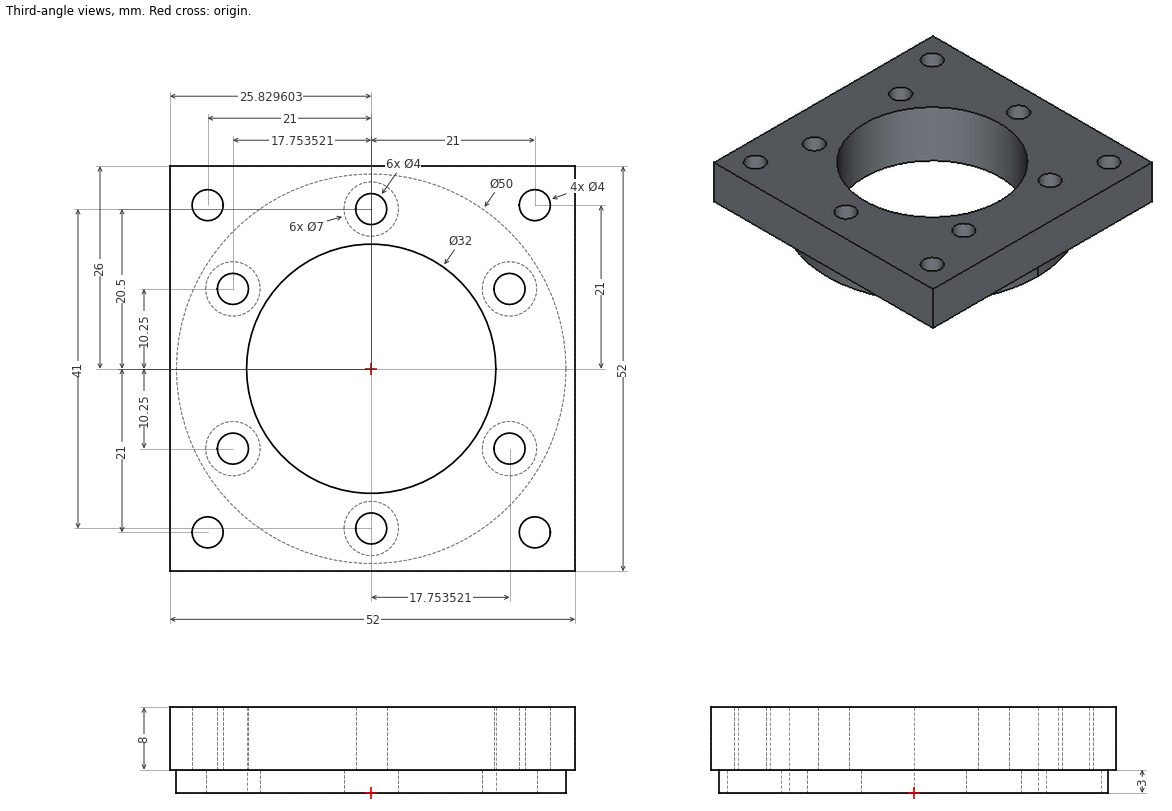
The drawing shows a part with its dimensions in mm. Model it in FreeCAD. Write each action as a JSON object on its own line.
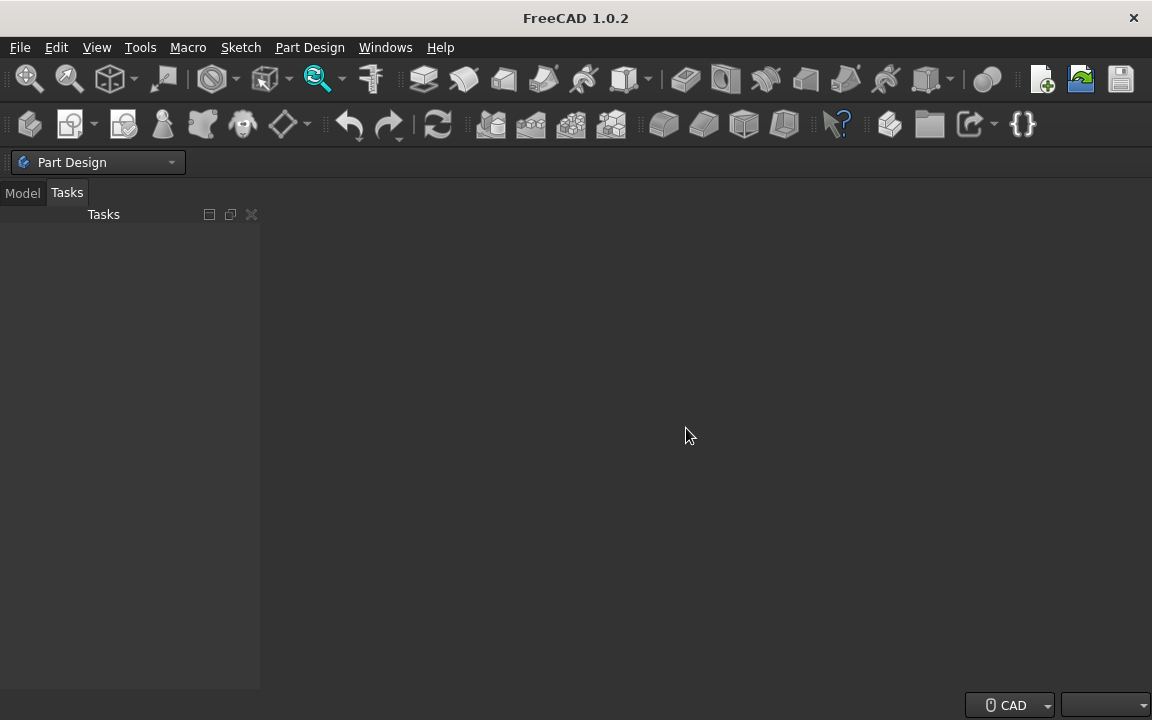
{"action": "key", "text": "ctrl+n"}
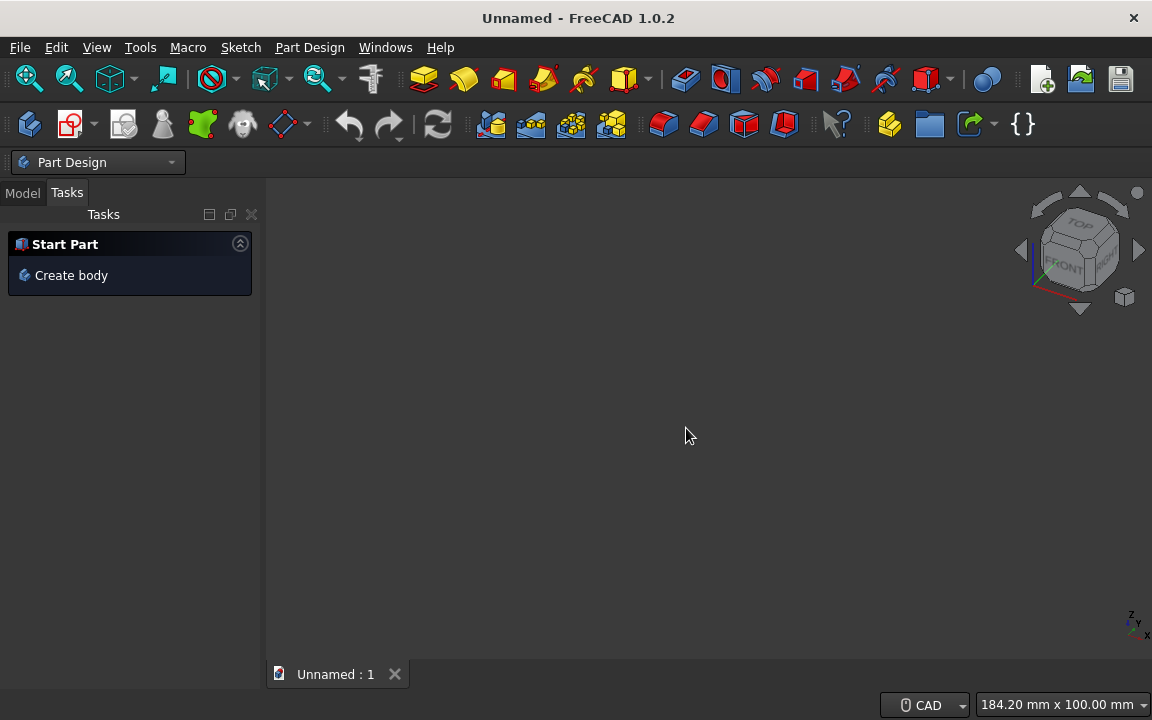
{"action": "left_click", "coordinate": [70, 124]}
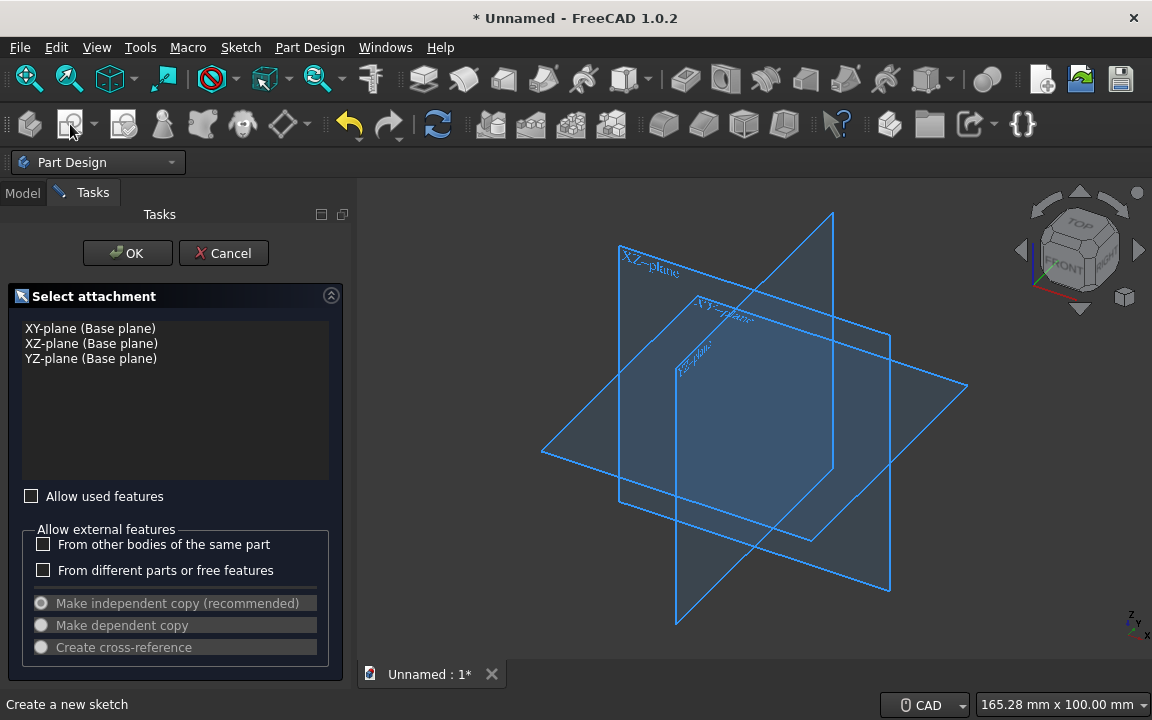
{"action": "left_click", "coordinate": [82, 328]}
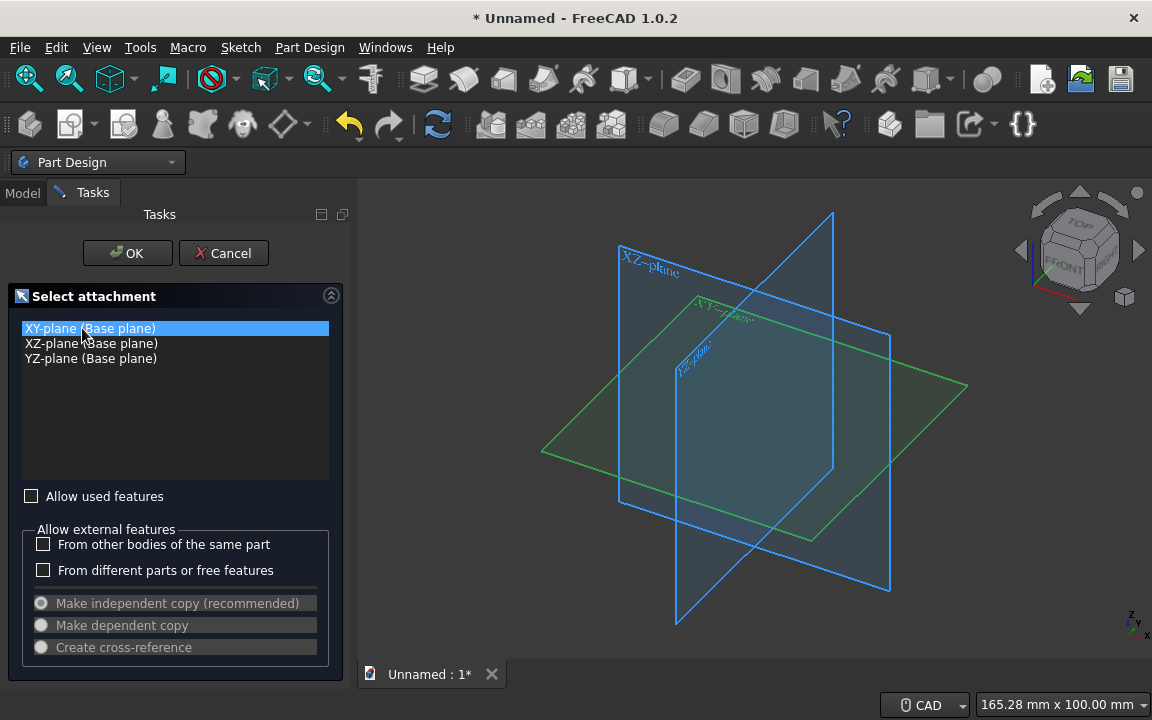
{"action": "left_click", "coordinate": [128, 253]}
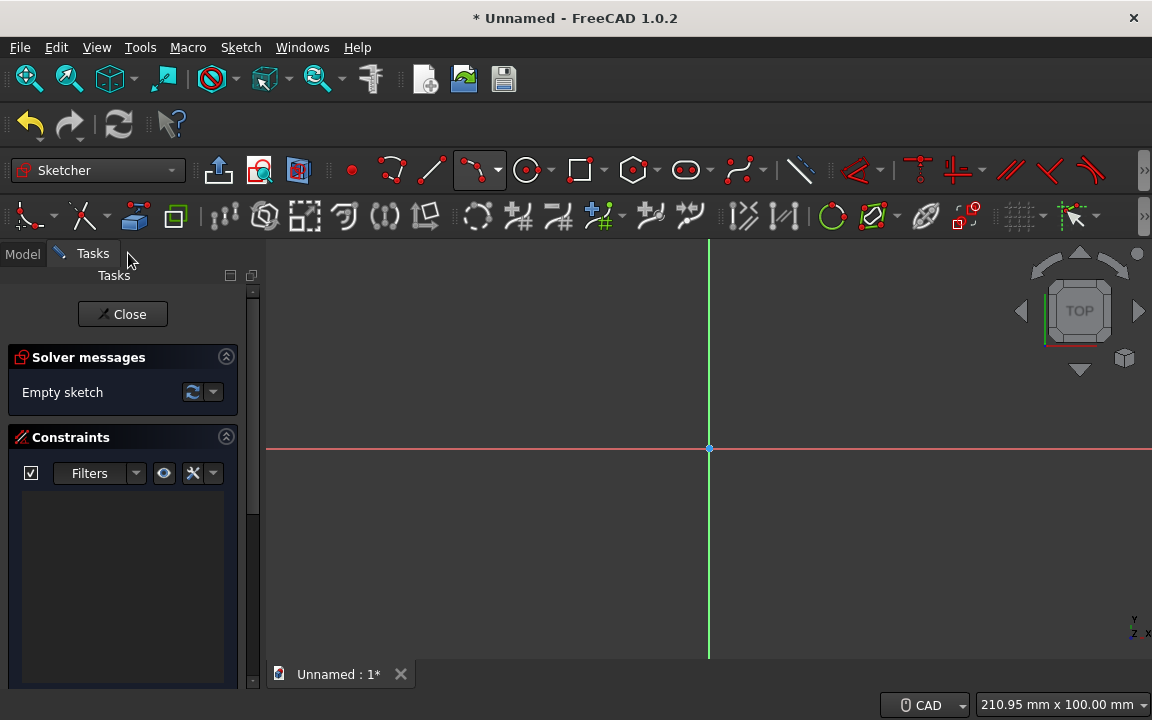
{"action": "key", "text": "g c"}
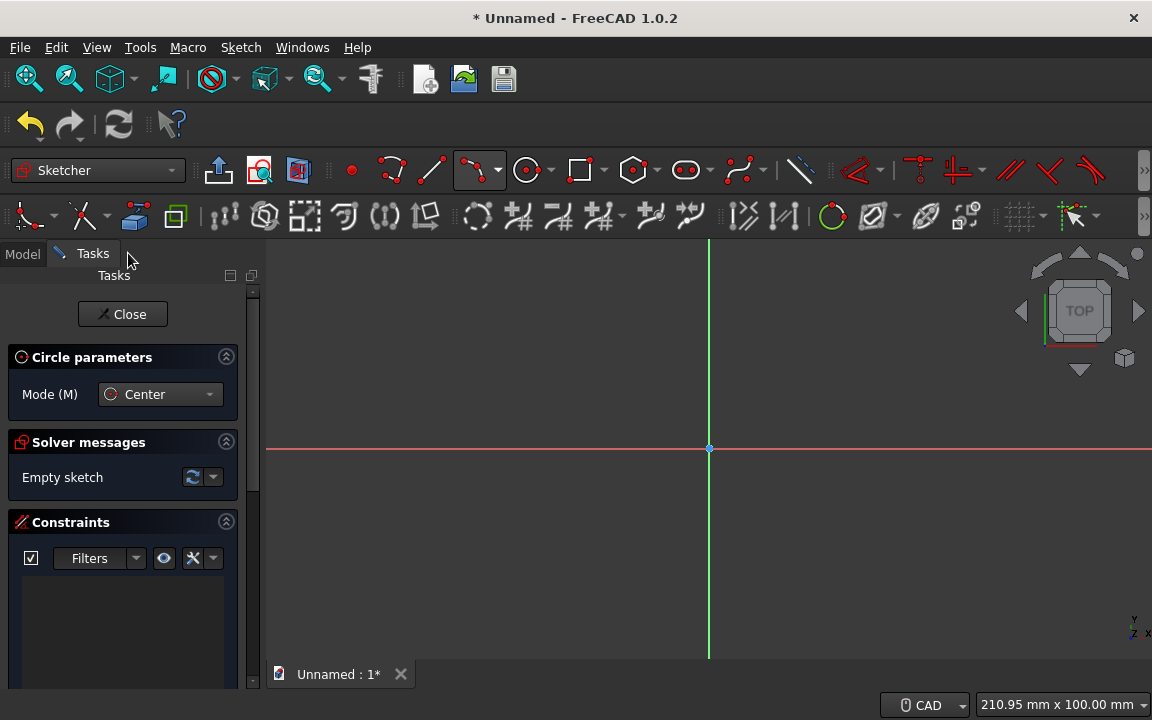
{"action": "left_click", "coordinate": [709, 449]}
{"action": "mouse_move", "coordinate": [783, 375]}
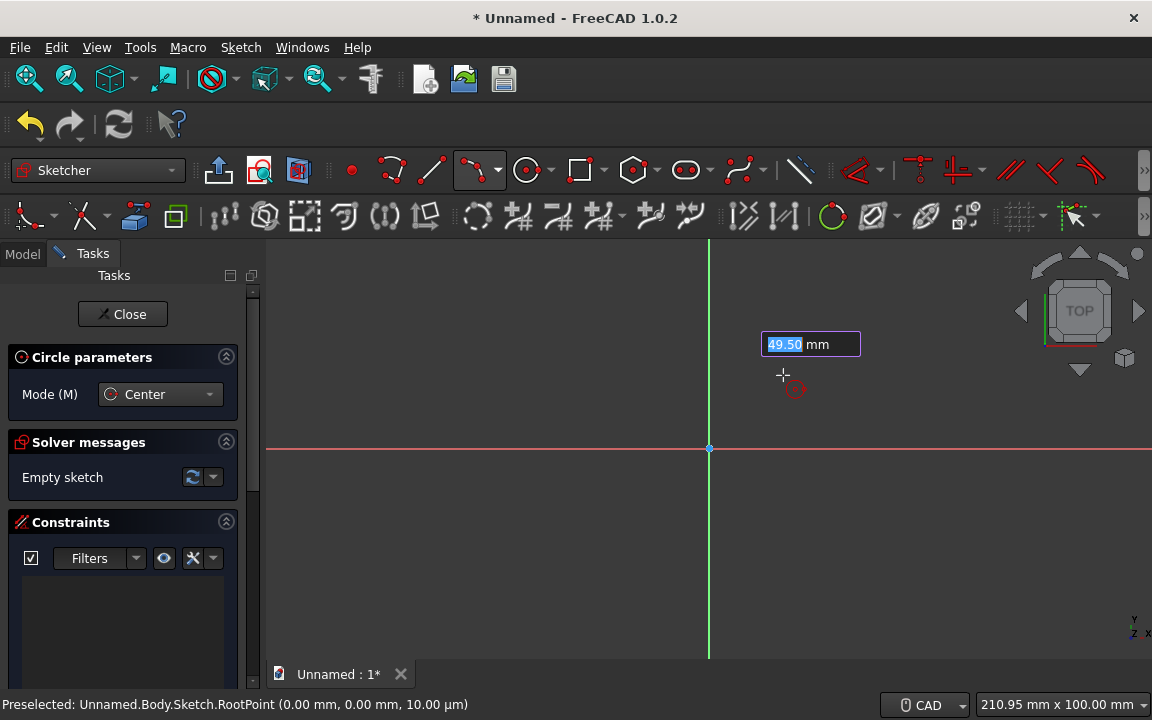
{"action": "type", "text": "50"}
{"action": "key", "text": "Return"}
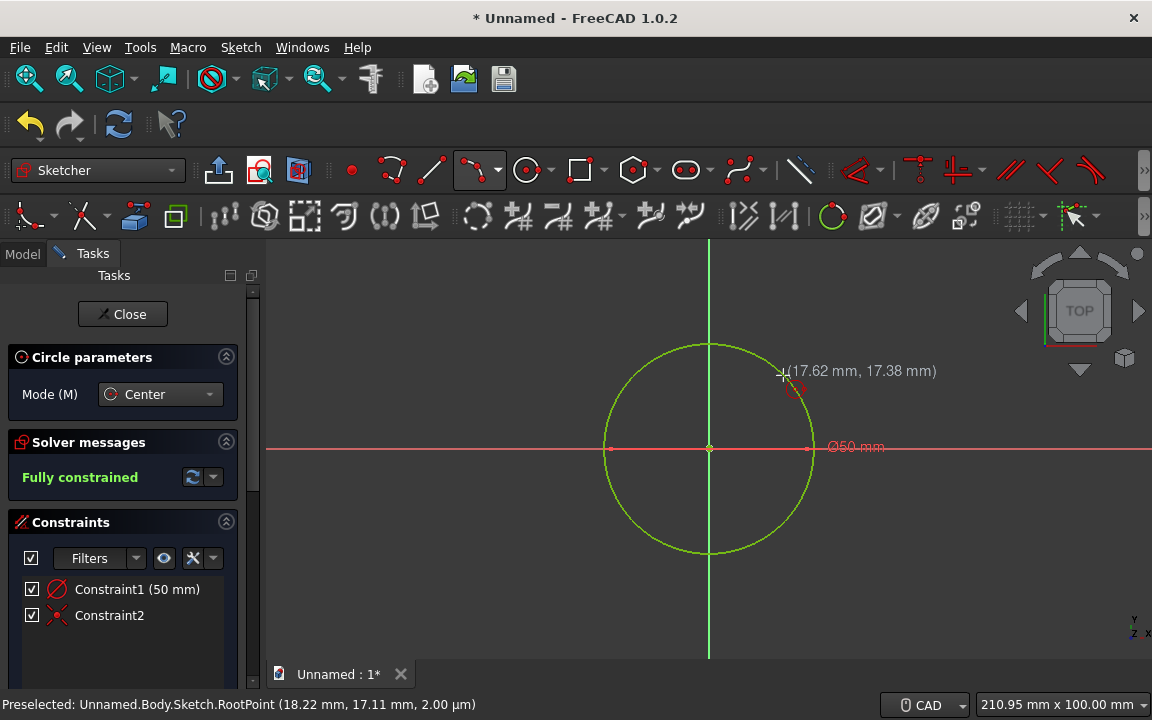
{"action": "left_click", "coordinate": [709, 449]}
{"action": "mouse_move", "coordinate": [757, 401]}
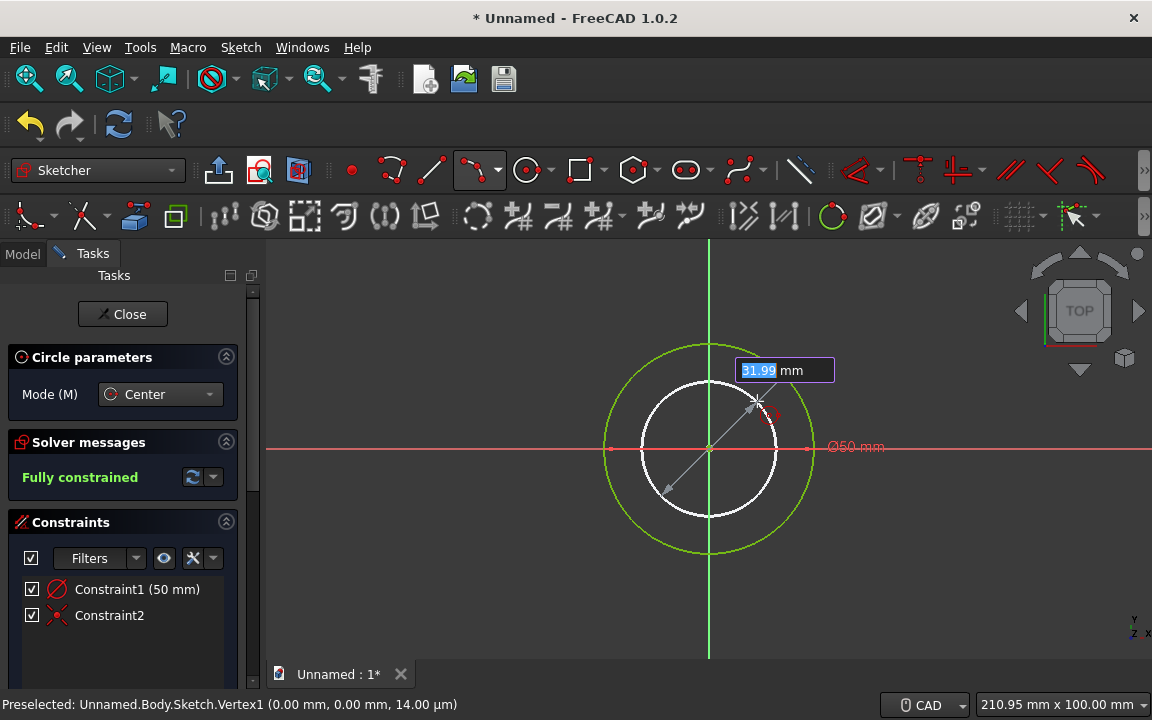
{"action": "type", "text": "32"}
{"action": "key", "text": "Return"}
{"action": "key", "text": "Escape"}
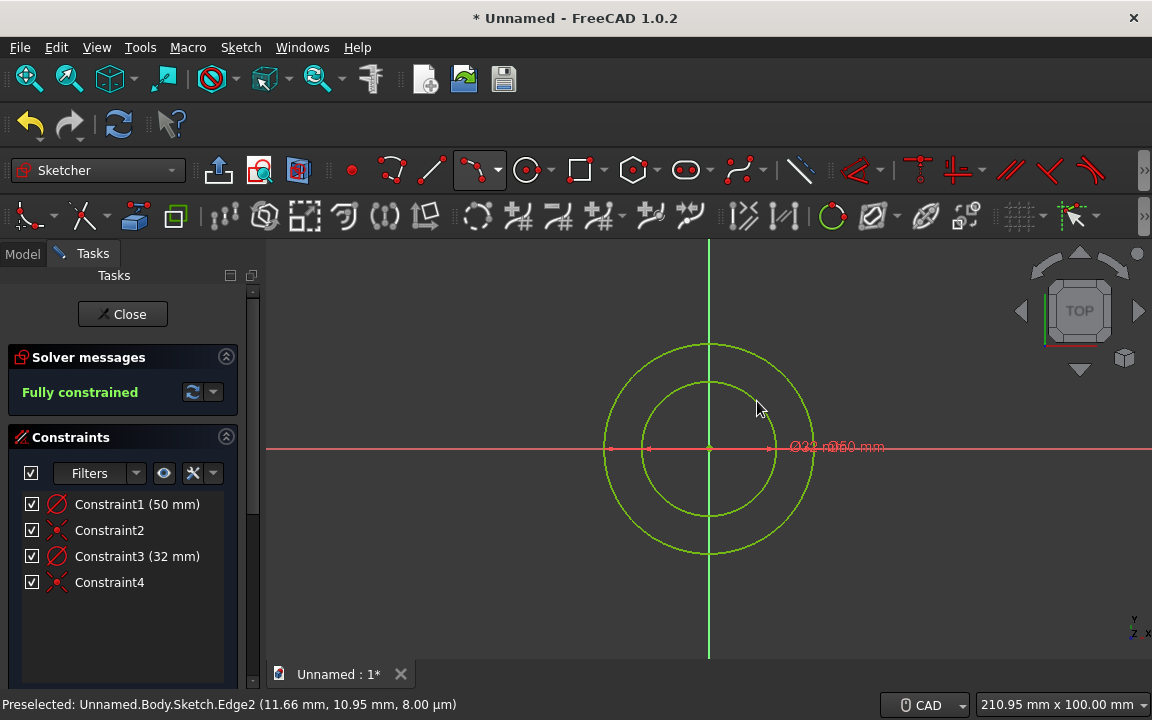
{"action": "left_click", "coordinate": [123, 314]}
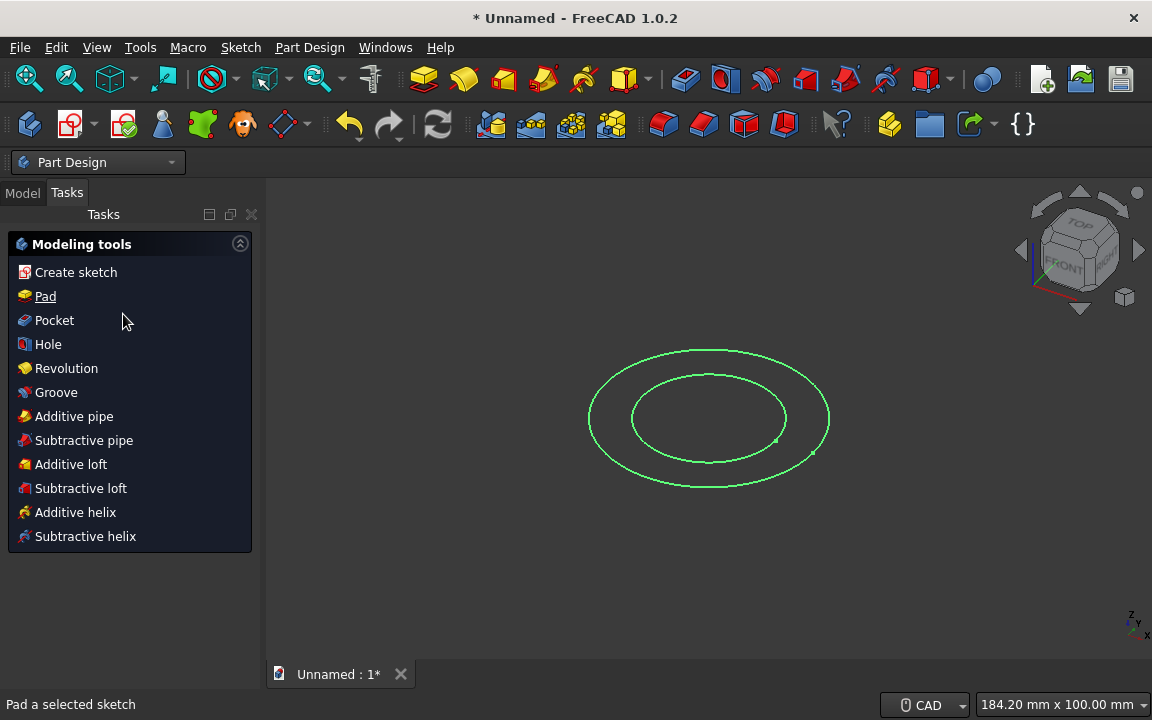
{"action": "left_click", "coordinate": [424, 80]}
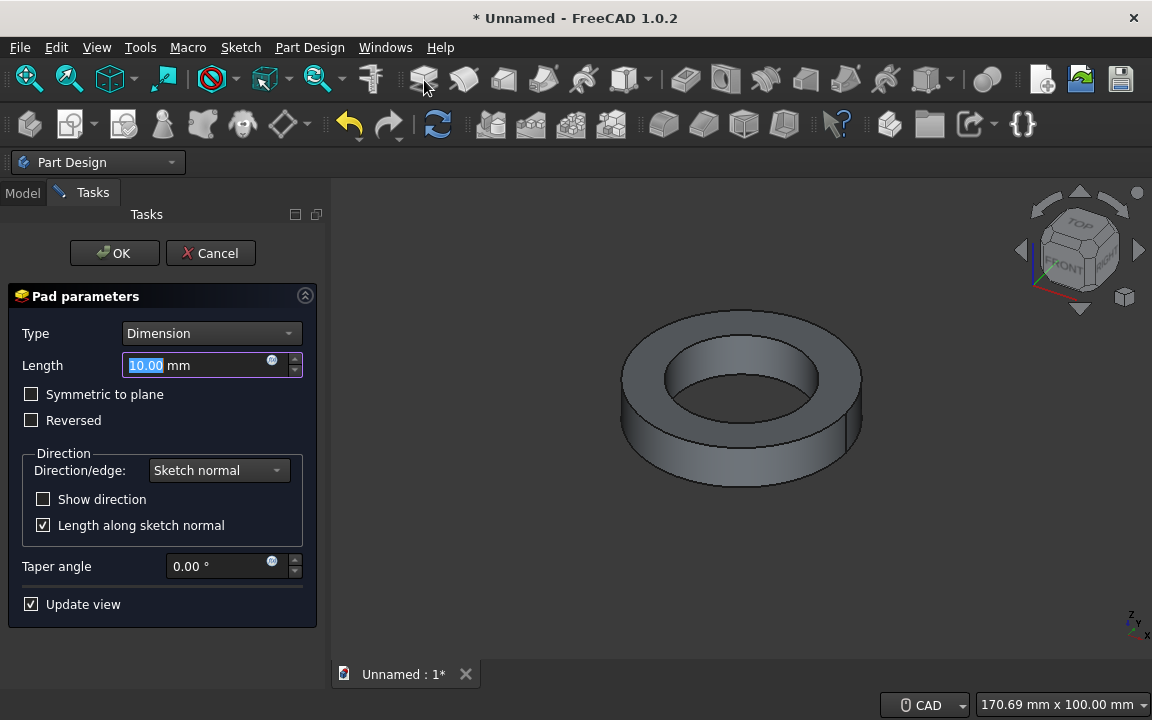
{"action": "type", "text": "3"}
{"action": "key", "text": "Tab"}